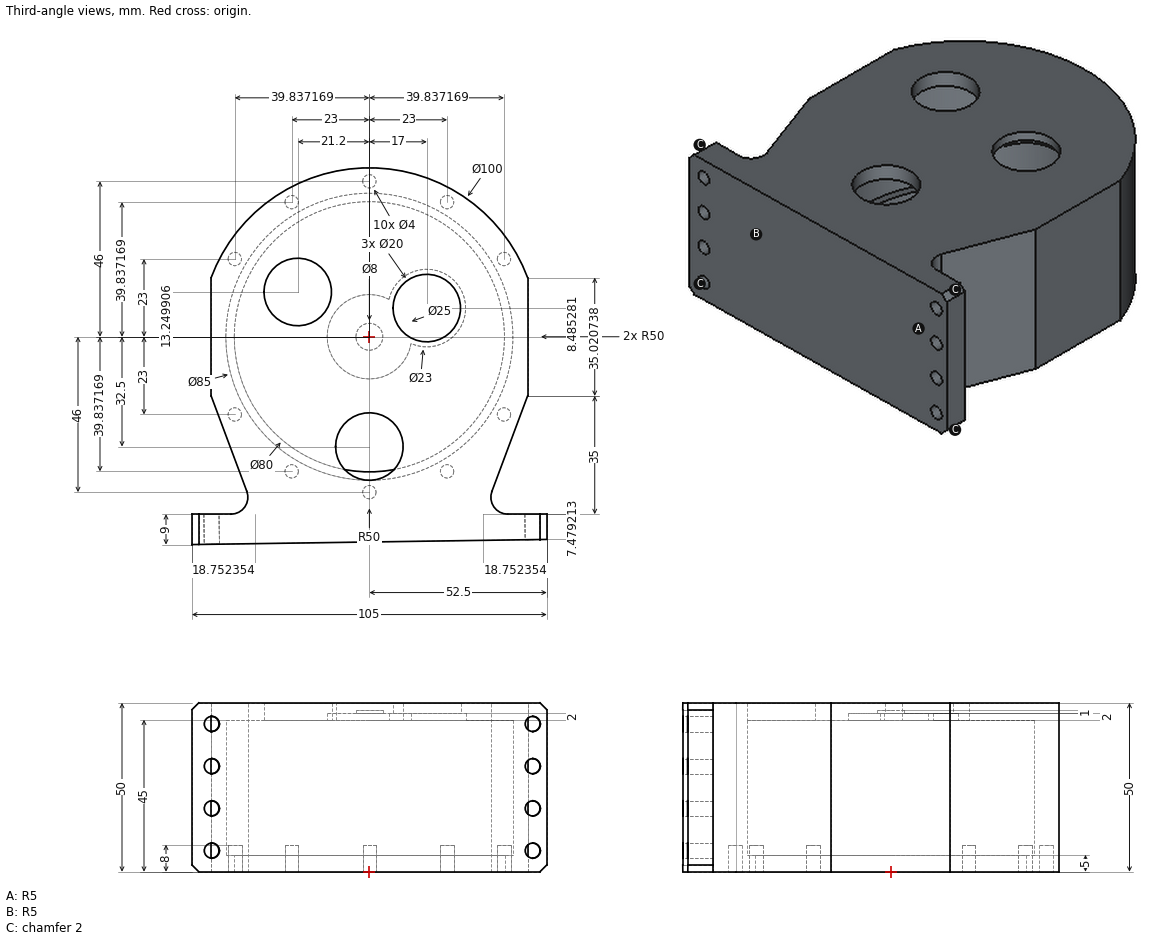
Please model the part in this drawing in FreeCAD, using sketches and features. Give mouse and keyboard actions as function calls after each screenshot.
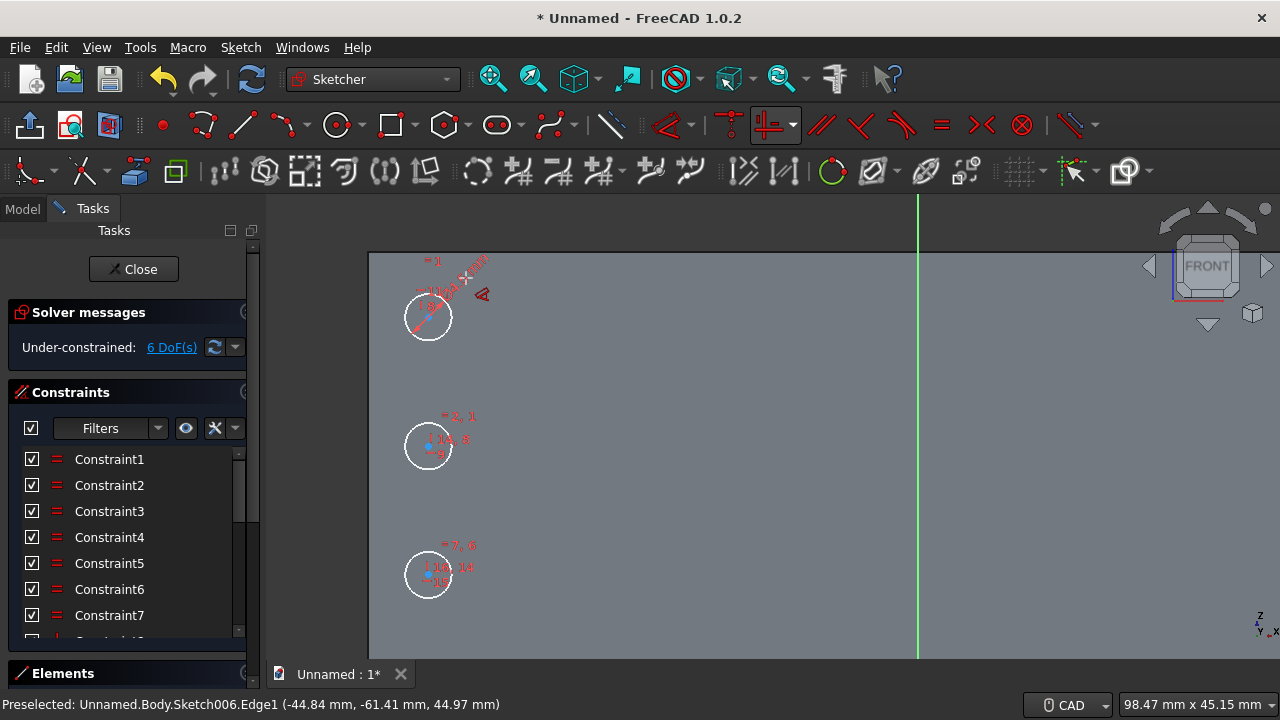
click(428, 446)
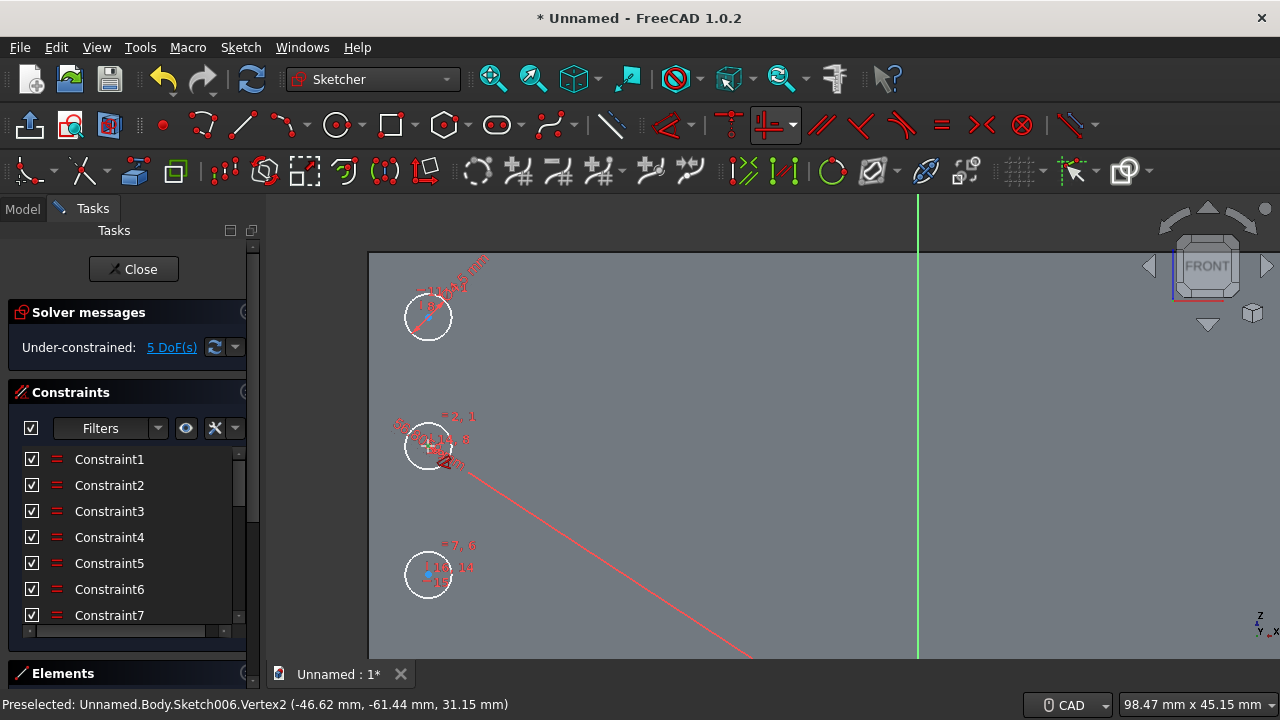
scroll(445, 300, down, 3)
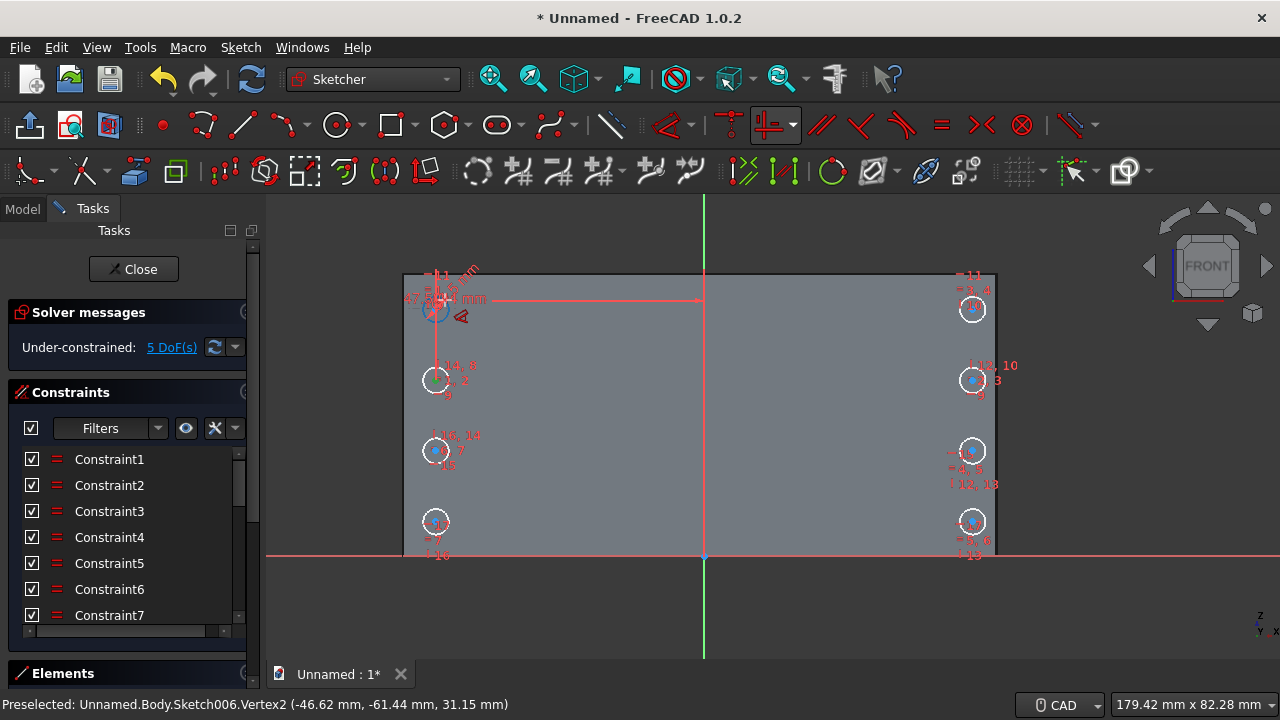
click(973, 380)
click(581, 346)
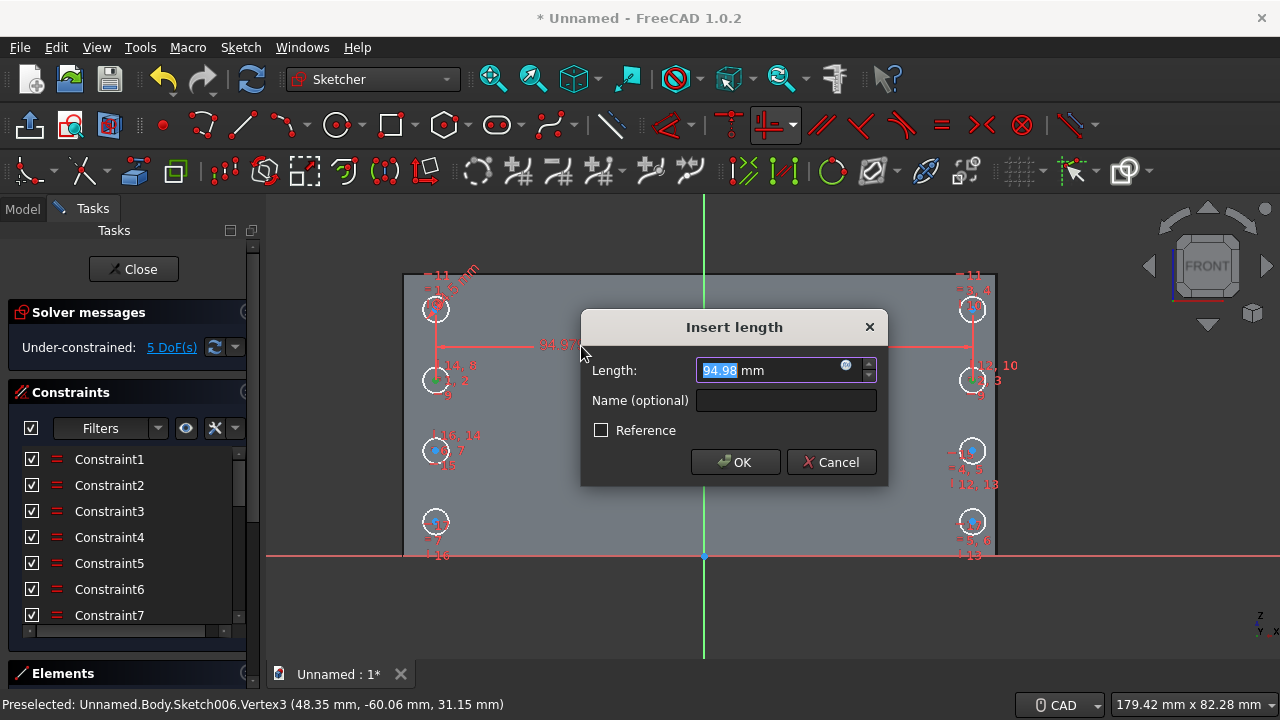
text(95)
key(Return)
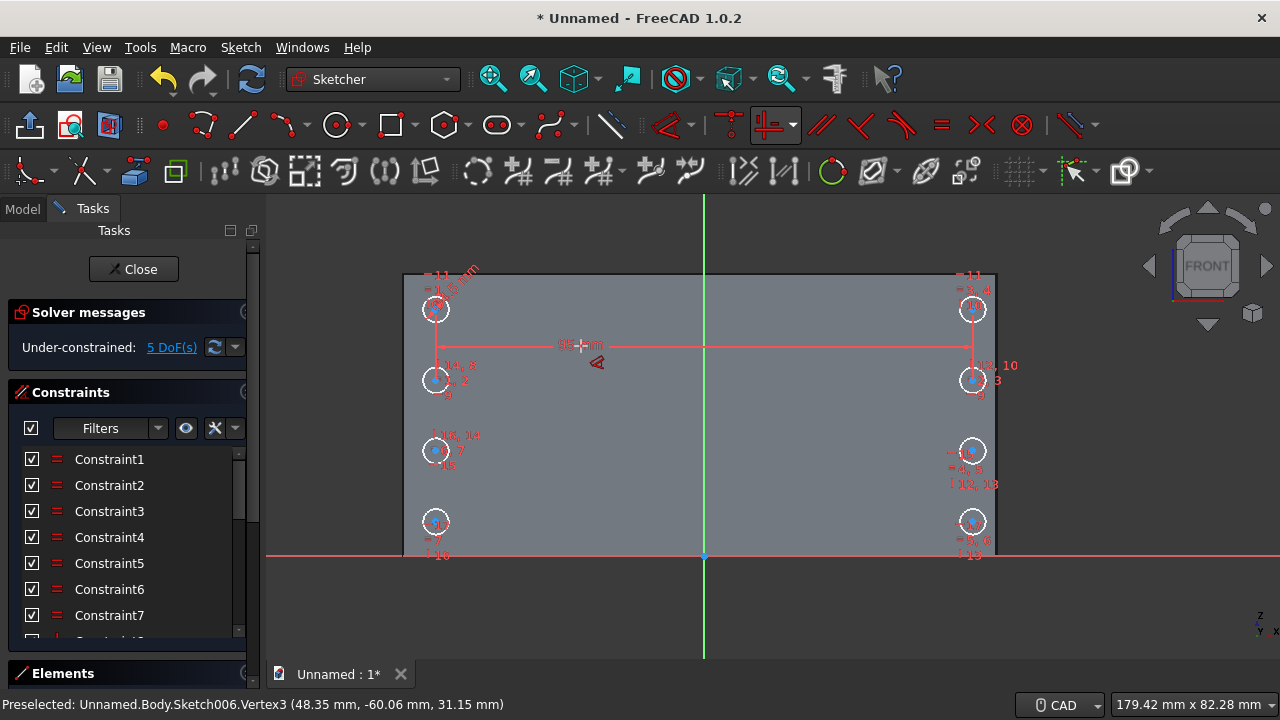
click(973, 310)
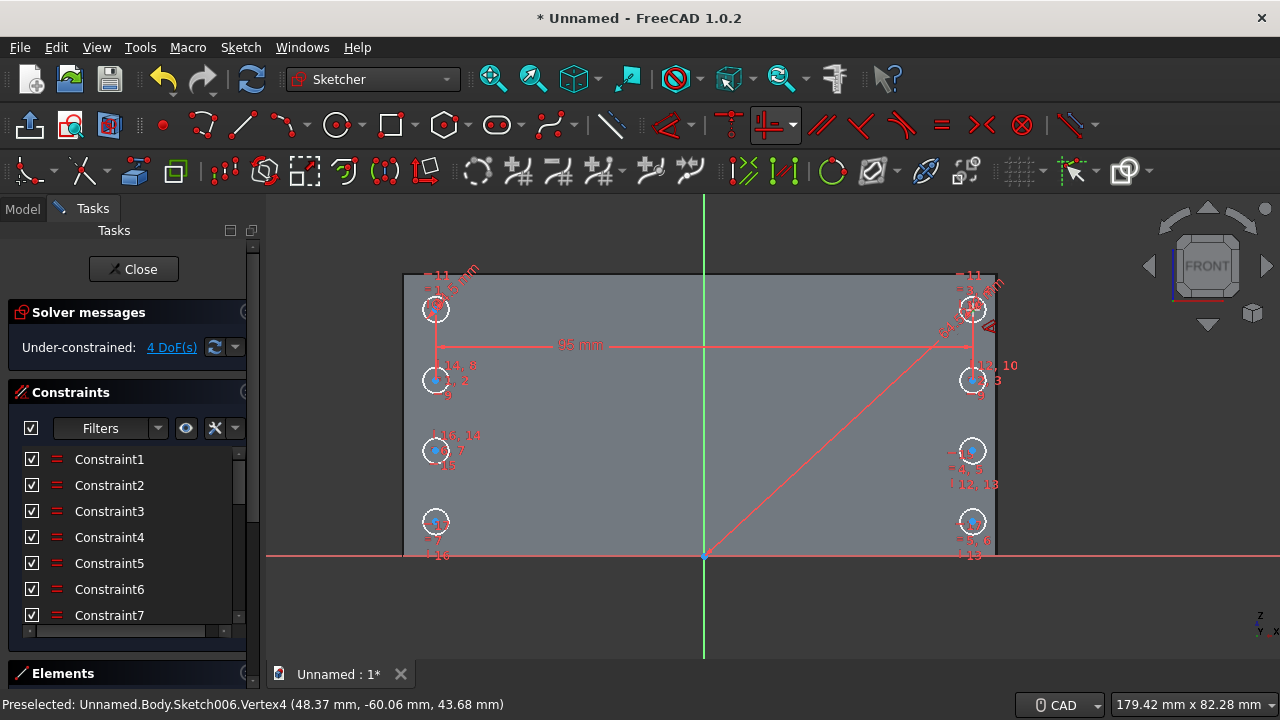
click(973, 451)
click(1007, 380)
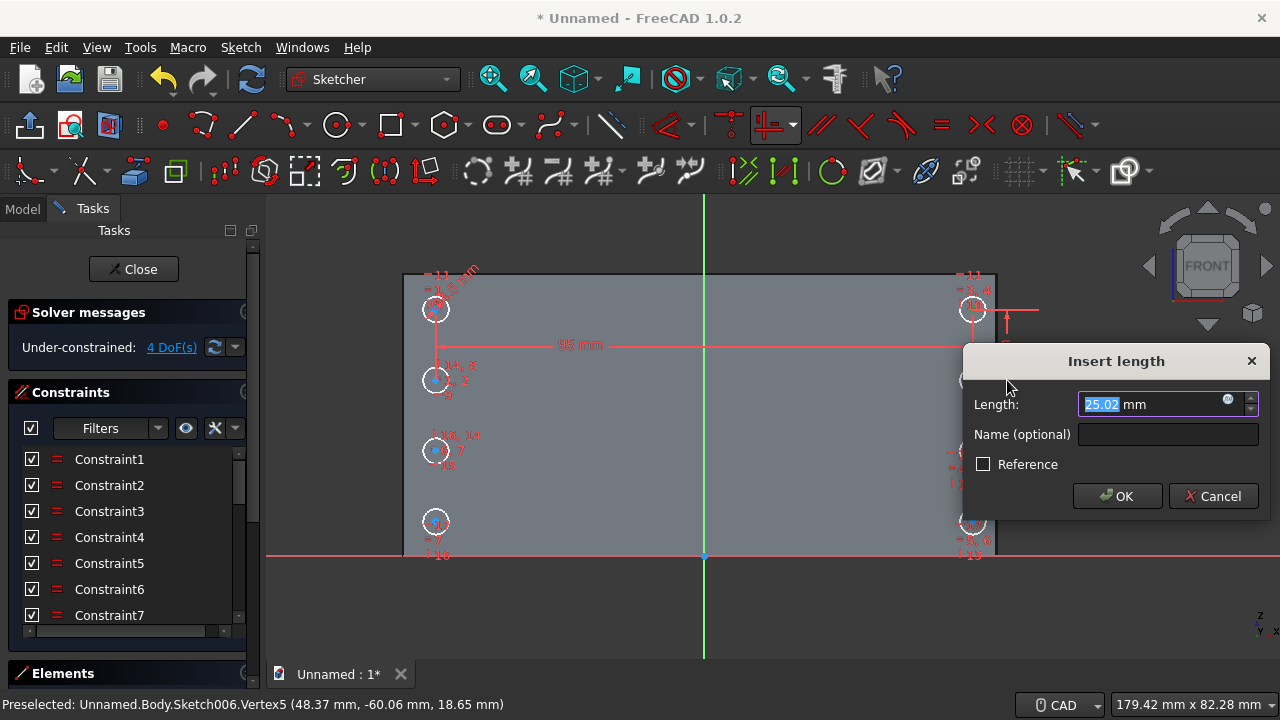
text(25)
key(Return)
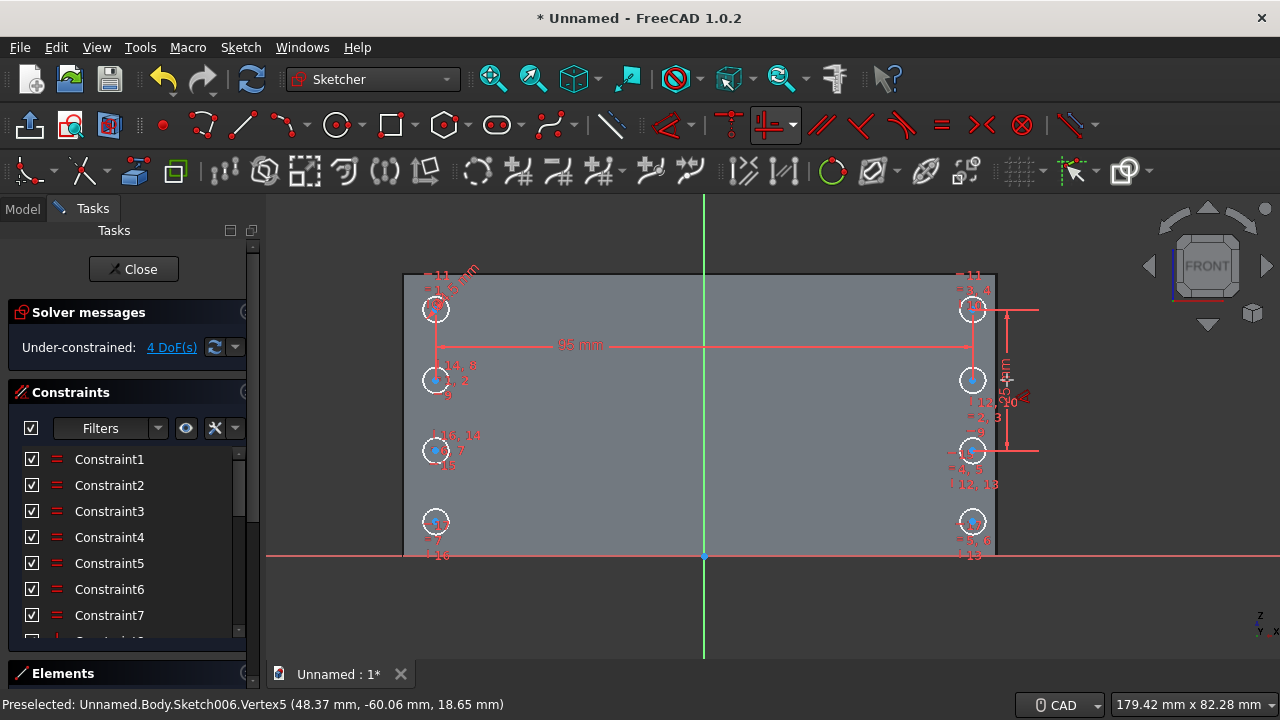
click(973, 380)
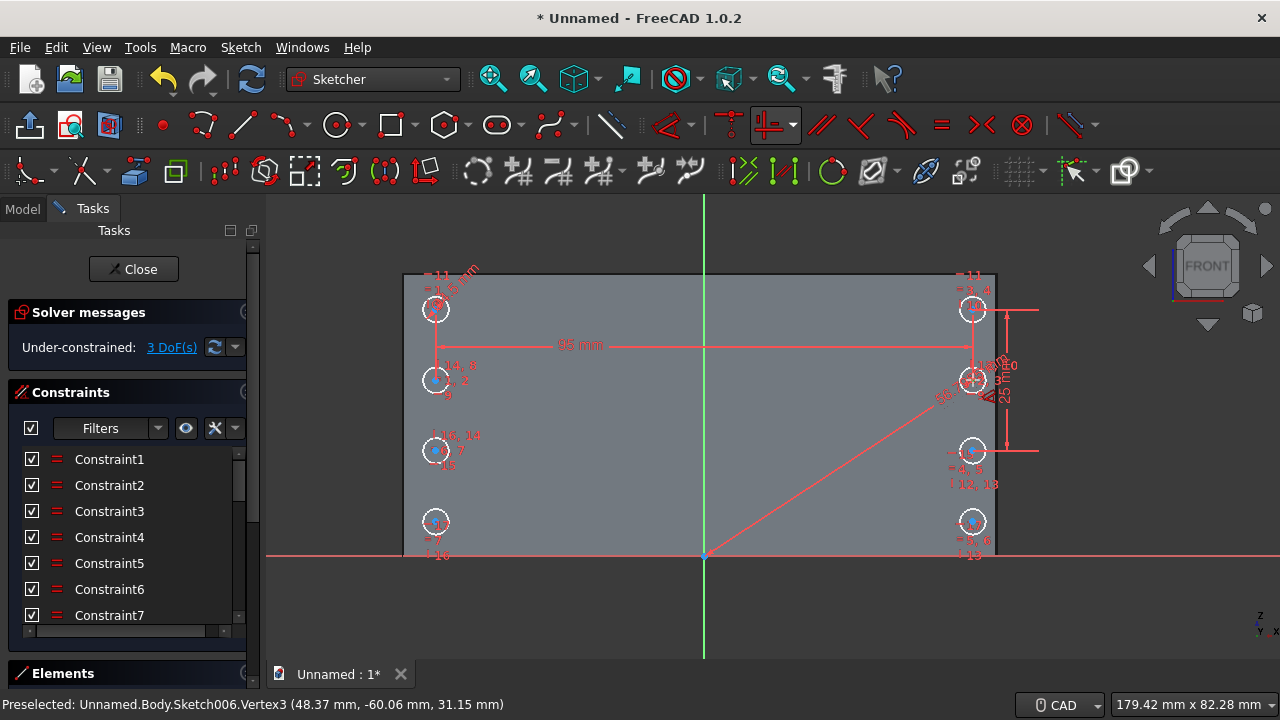
click(973, 522)
click(1007, 451)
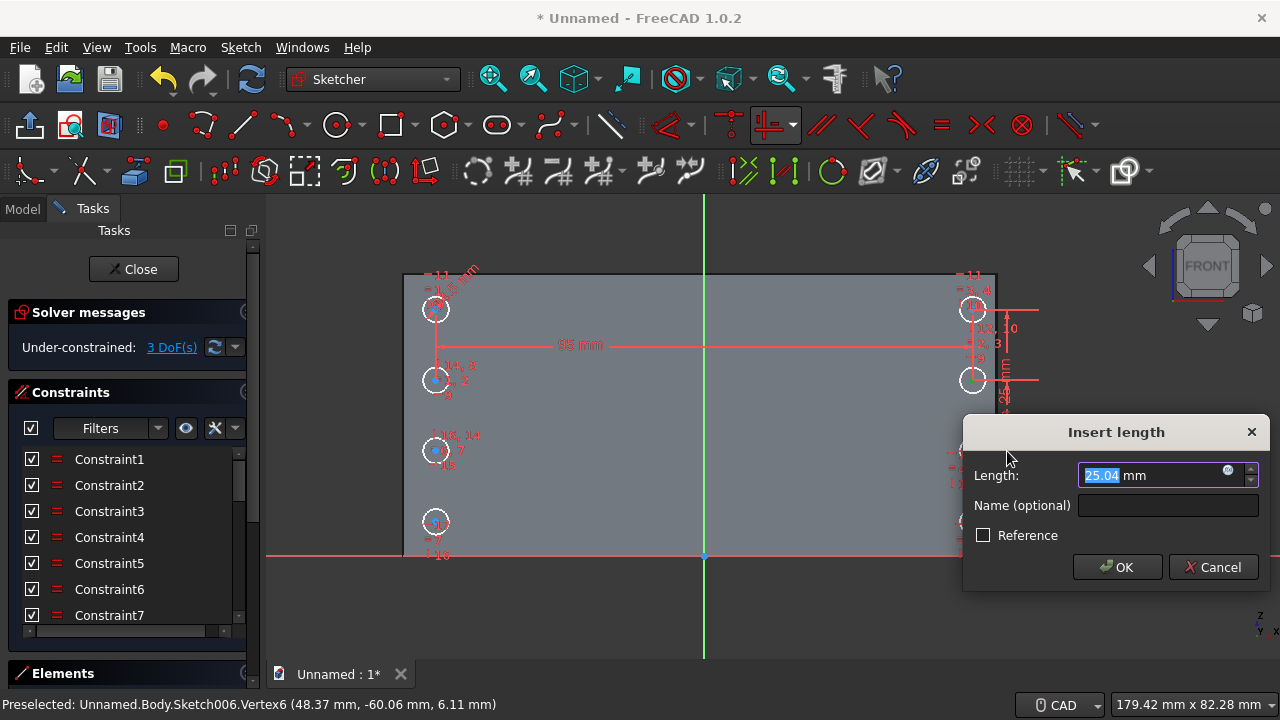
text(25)
key(Return)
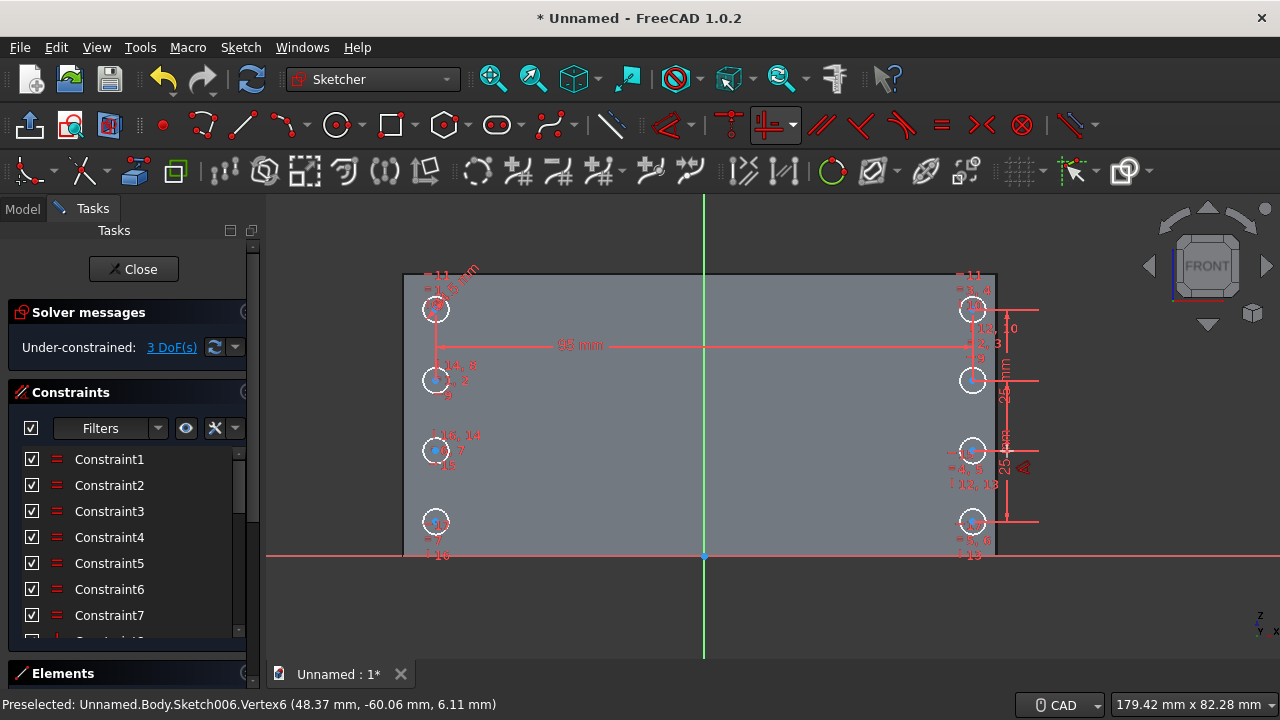
click(436, 310)
click(570, 590)